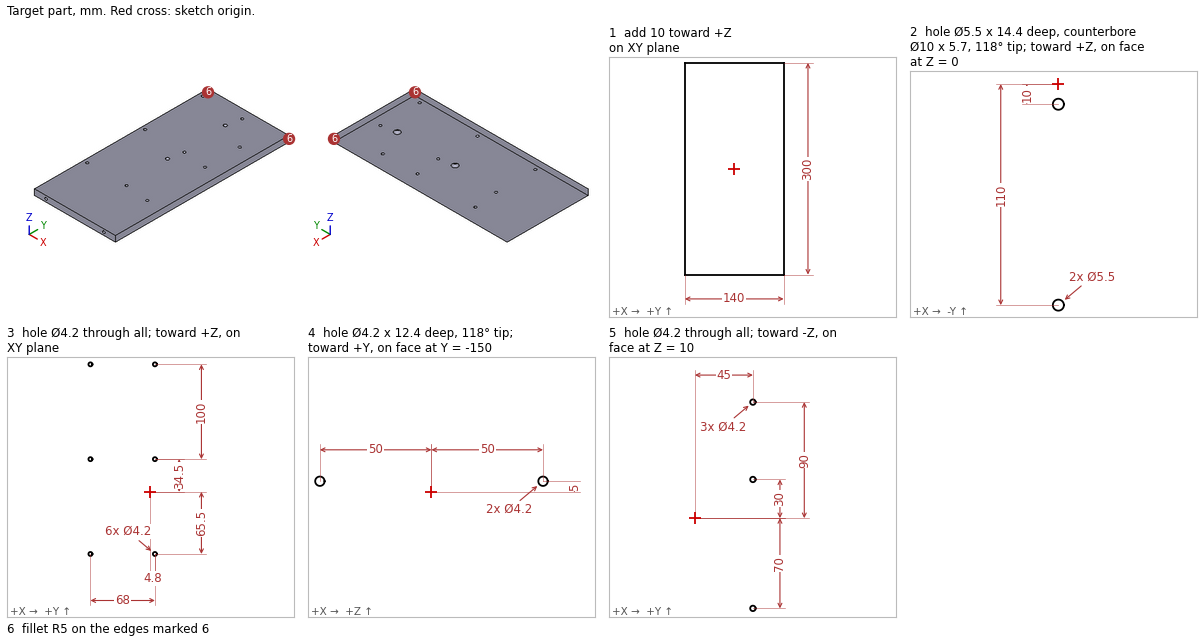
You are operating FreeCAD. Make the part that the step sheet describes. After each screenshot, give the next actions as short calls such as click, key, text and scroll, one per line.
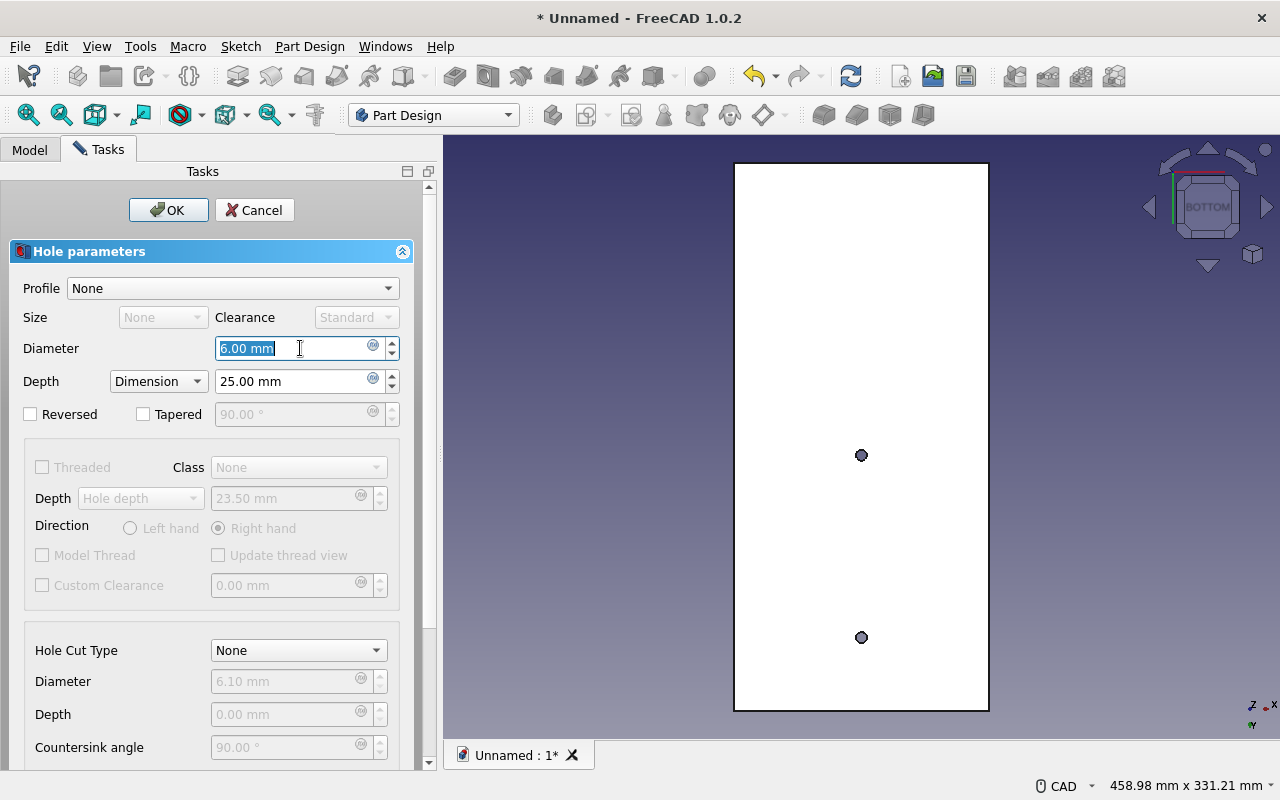
text(5.5)
key(Tab)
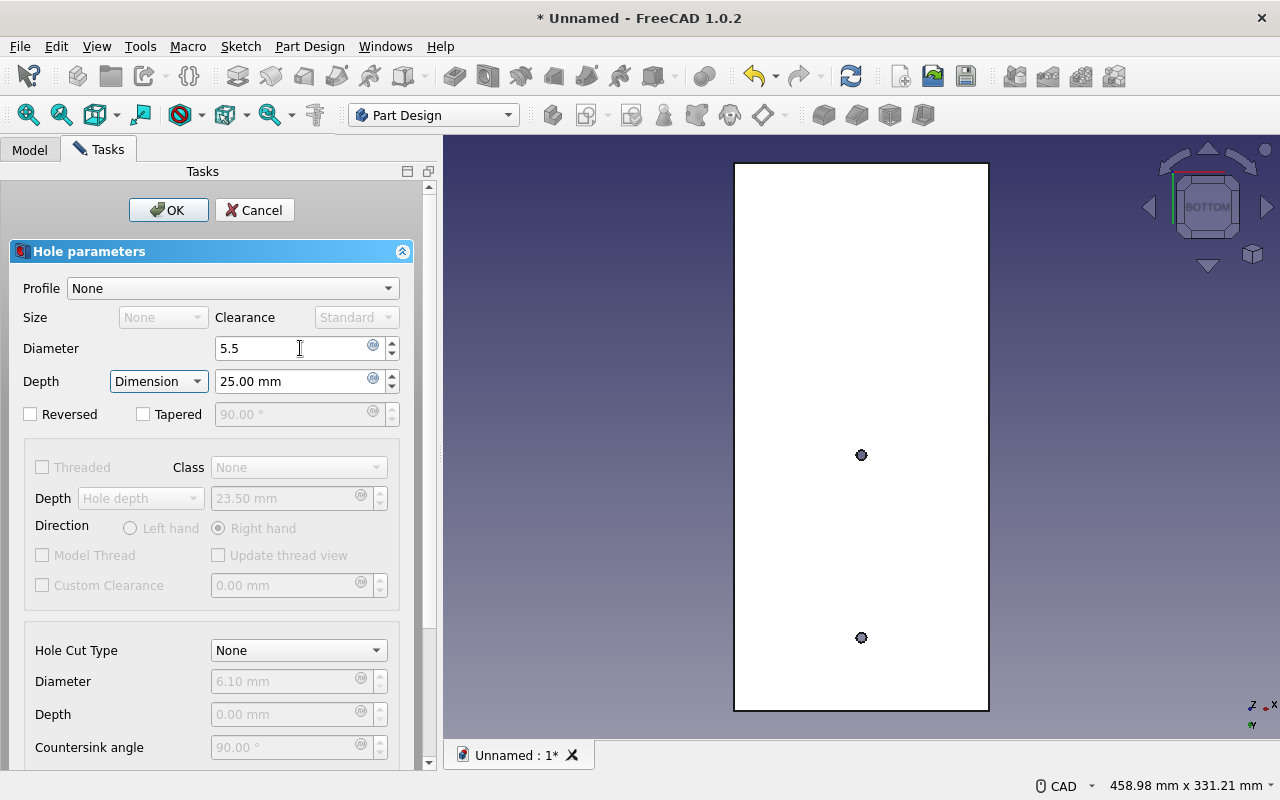
triple_click(300, 382)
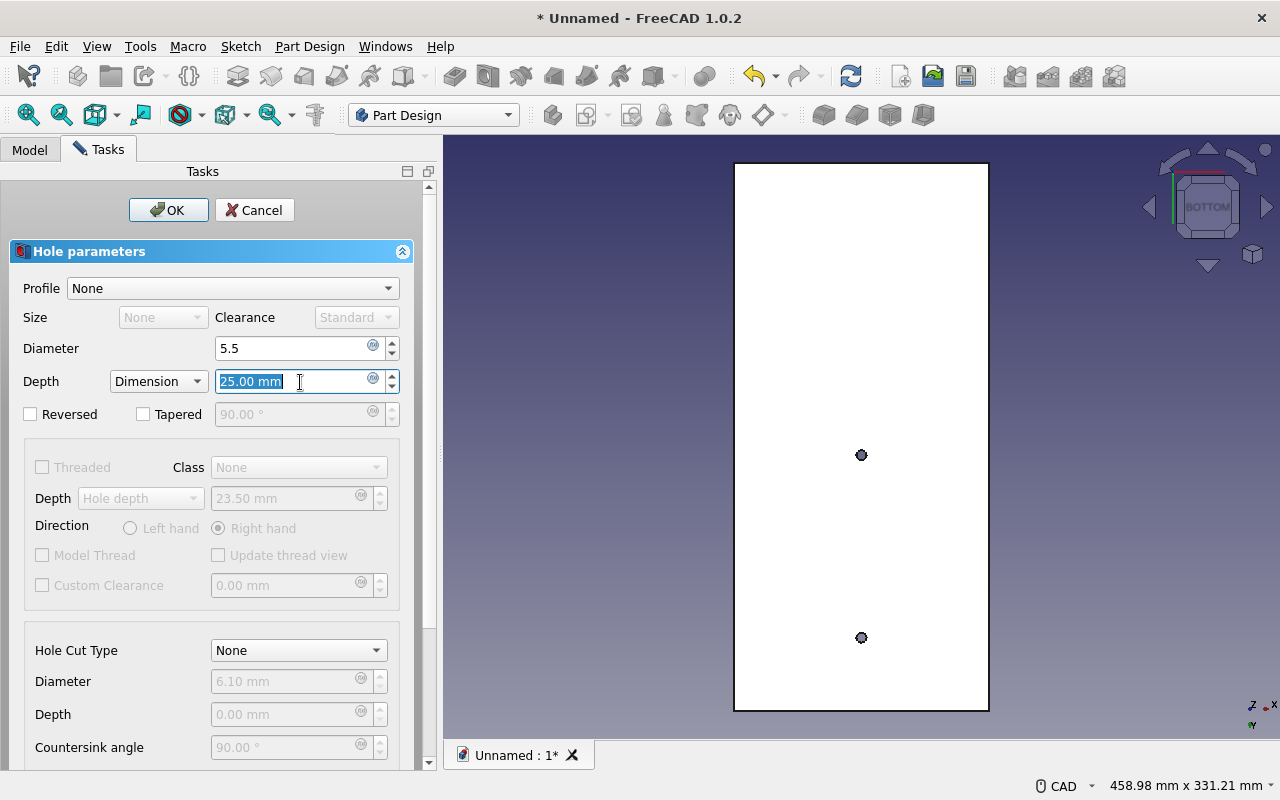
text(14.4)
key(Tab)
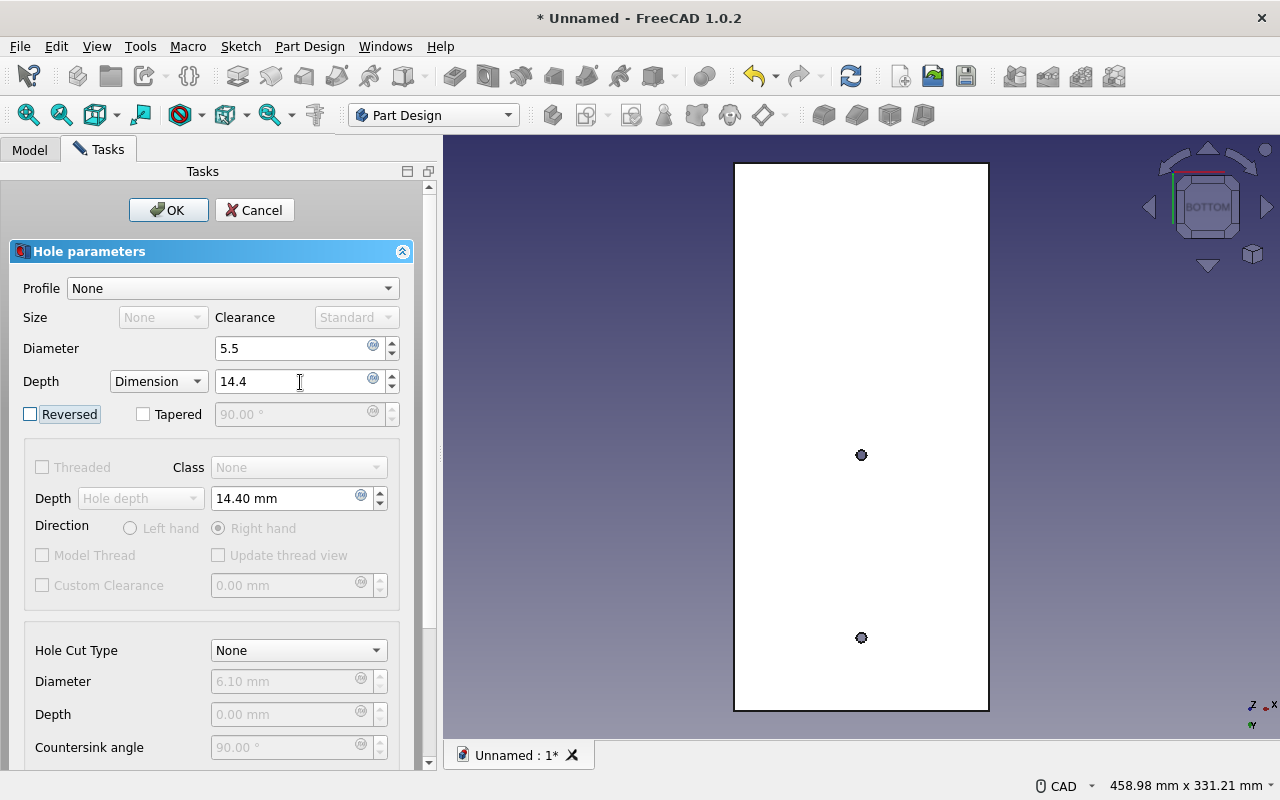
click(300, 650)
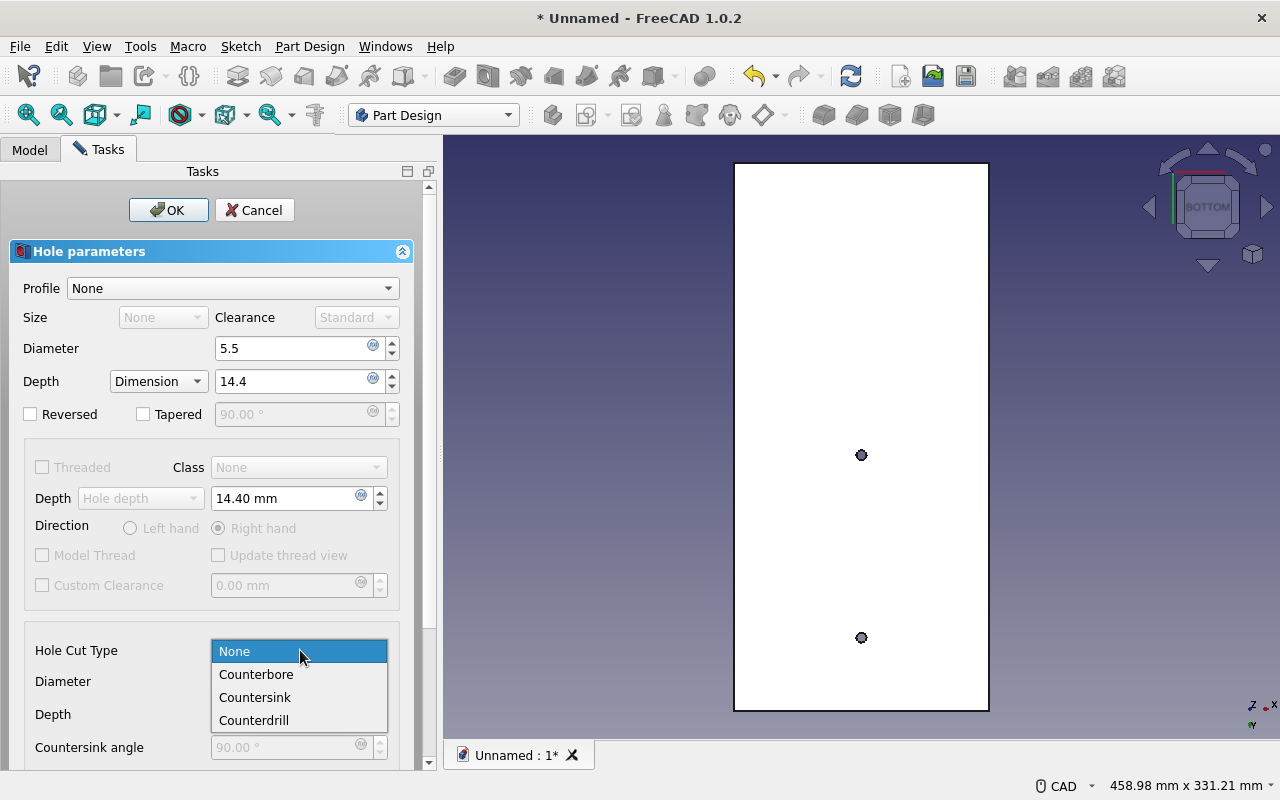
click(298, 674)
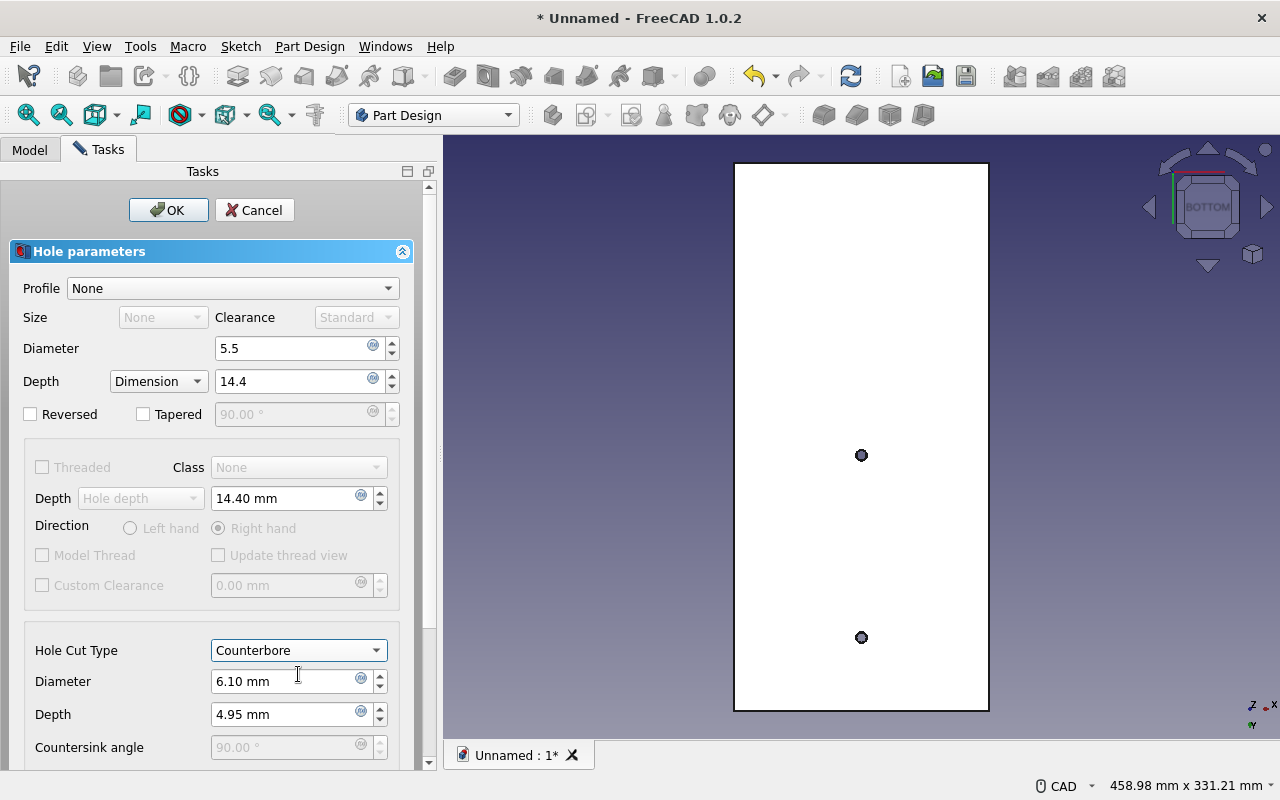
triple_click(292, 682)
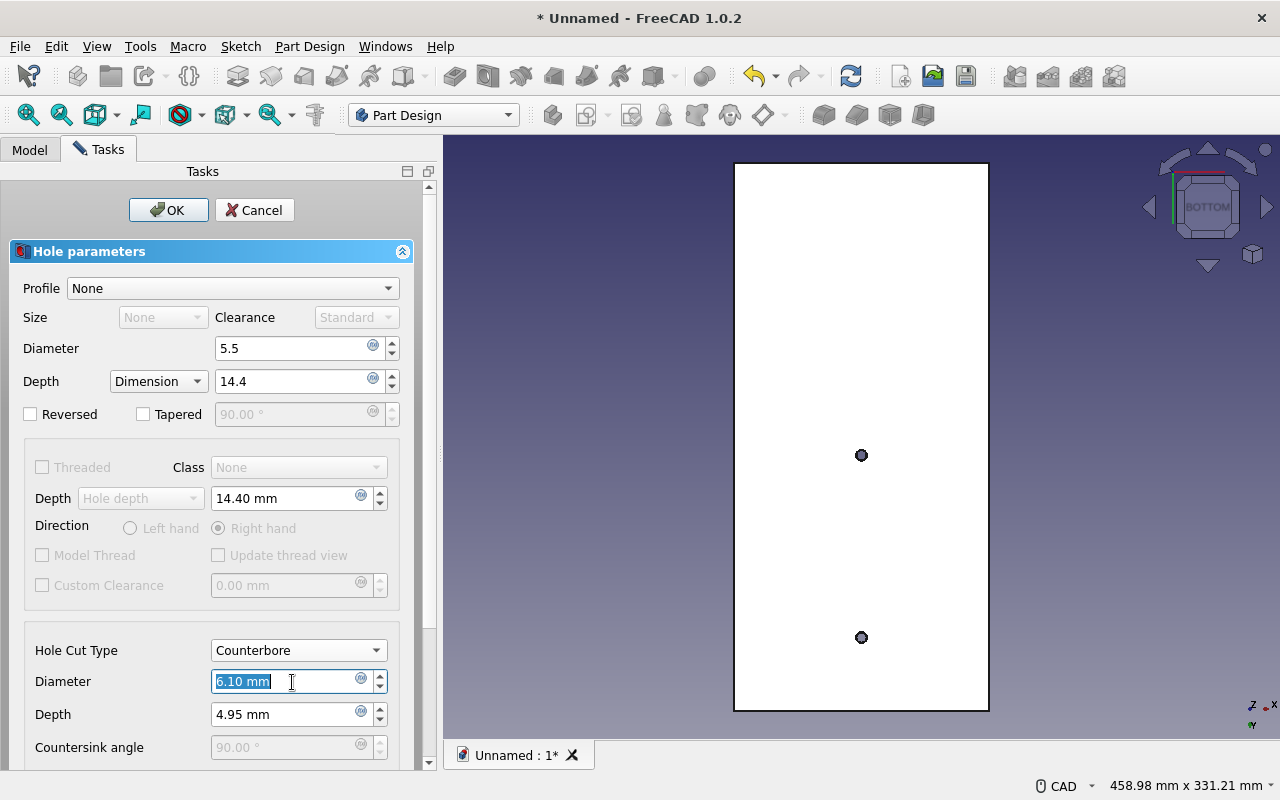
text(10)
key(Tab)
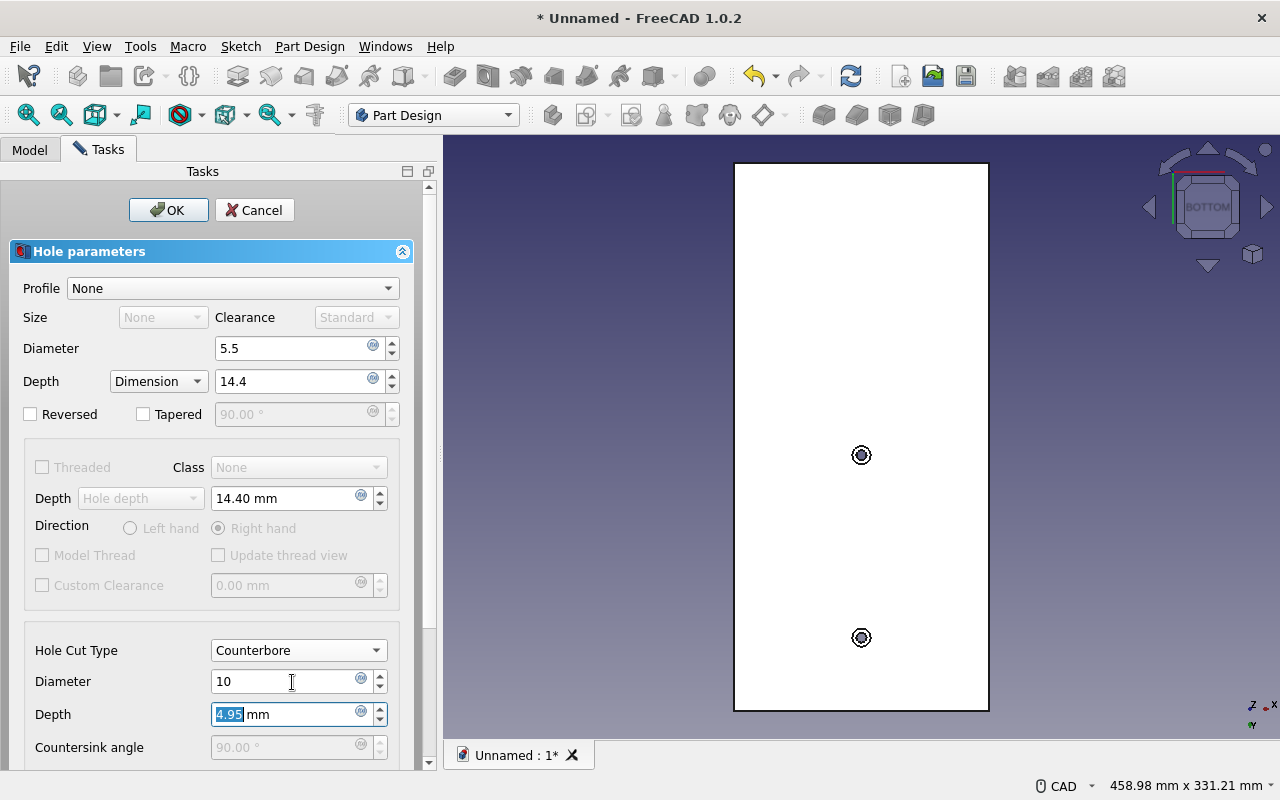
text(5.7)
key(Tab)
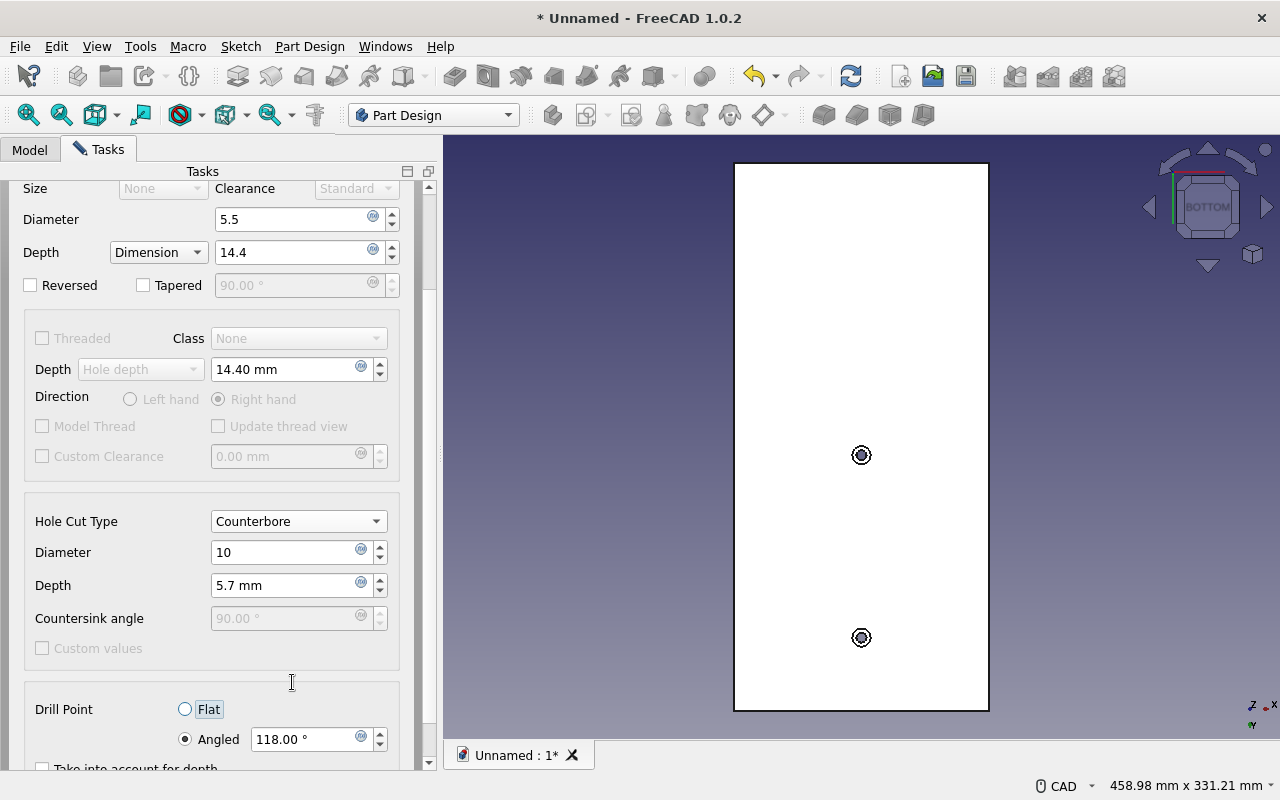
scroll(429, 476, up, 3)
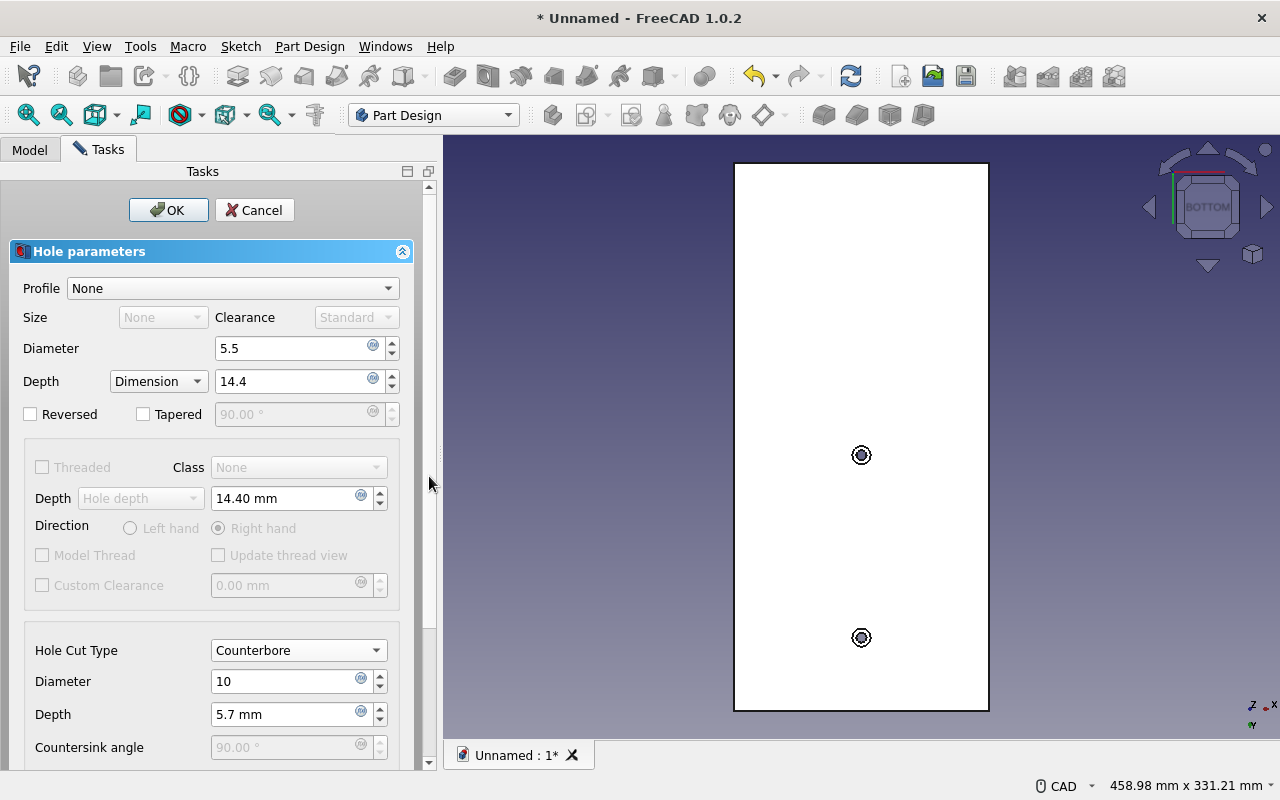
click(169, 210)